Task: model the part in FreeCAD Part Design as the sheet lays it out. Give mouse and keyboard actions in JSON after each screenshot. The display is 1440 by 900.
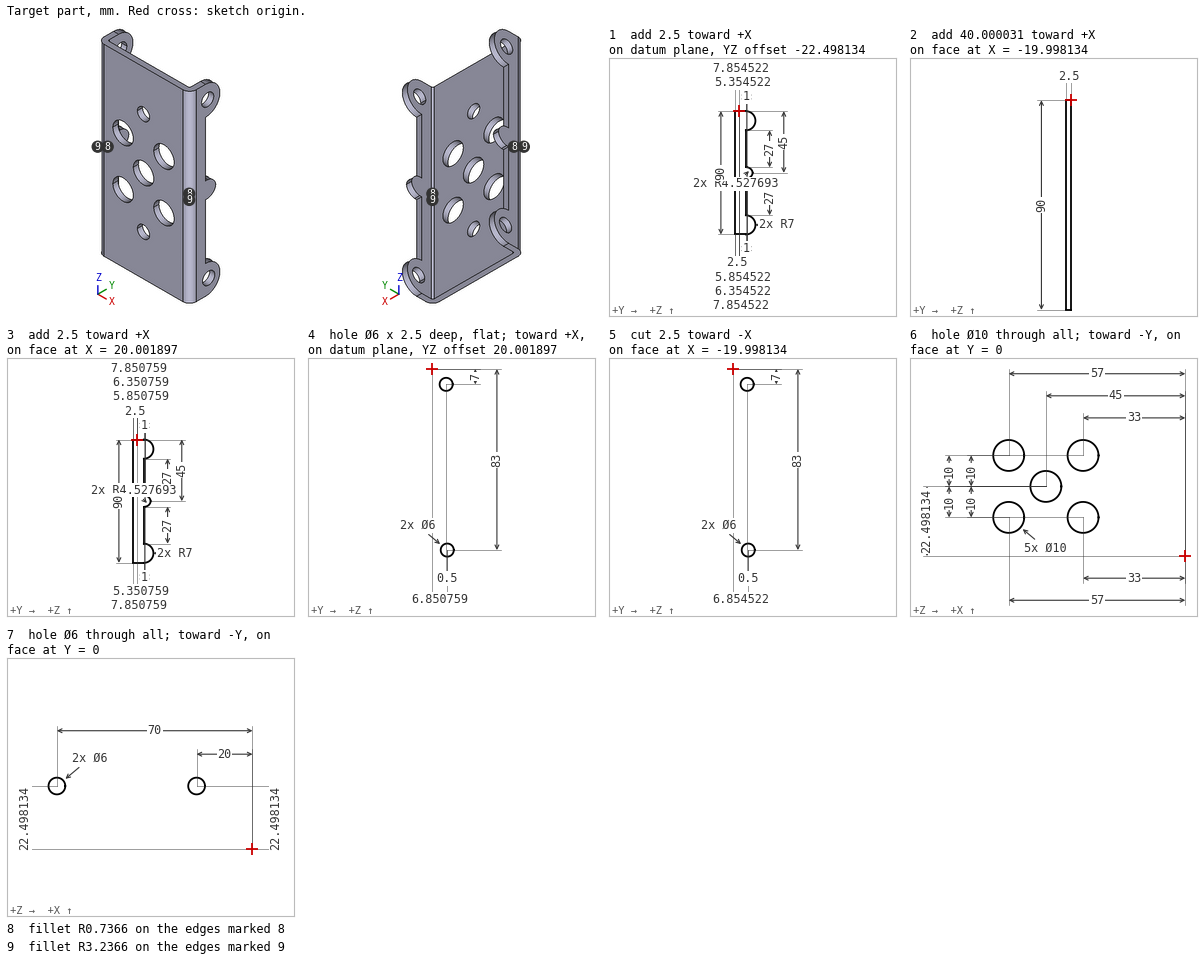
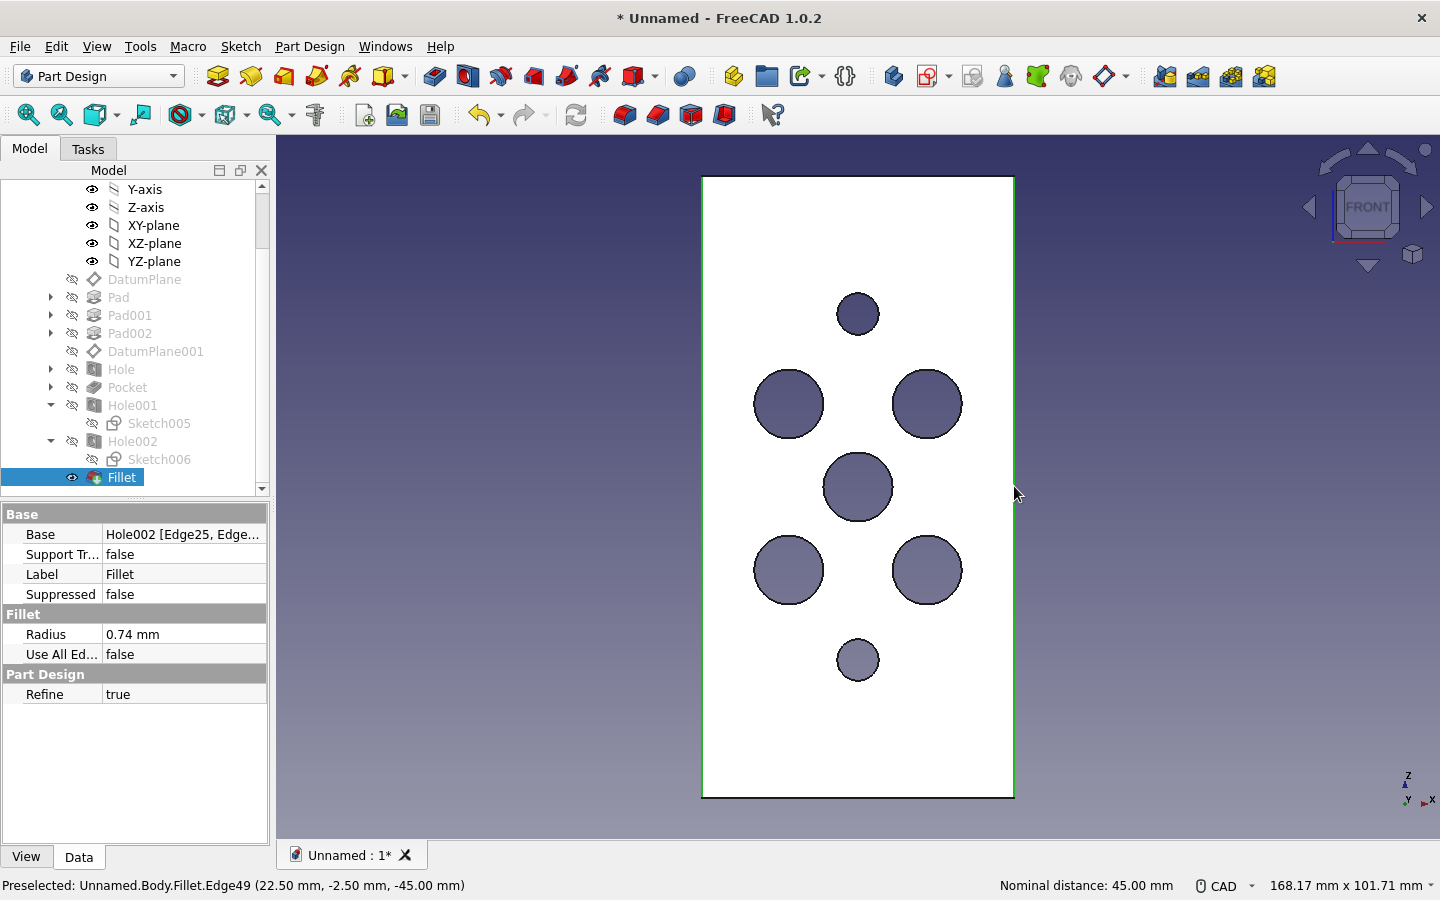
{"action": "left_click", "coordinate": [625, 116]}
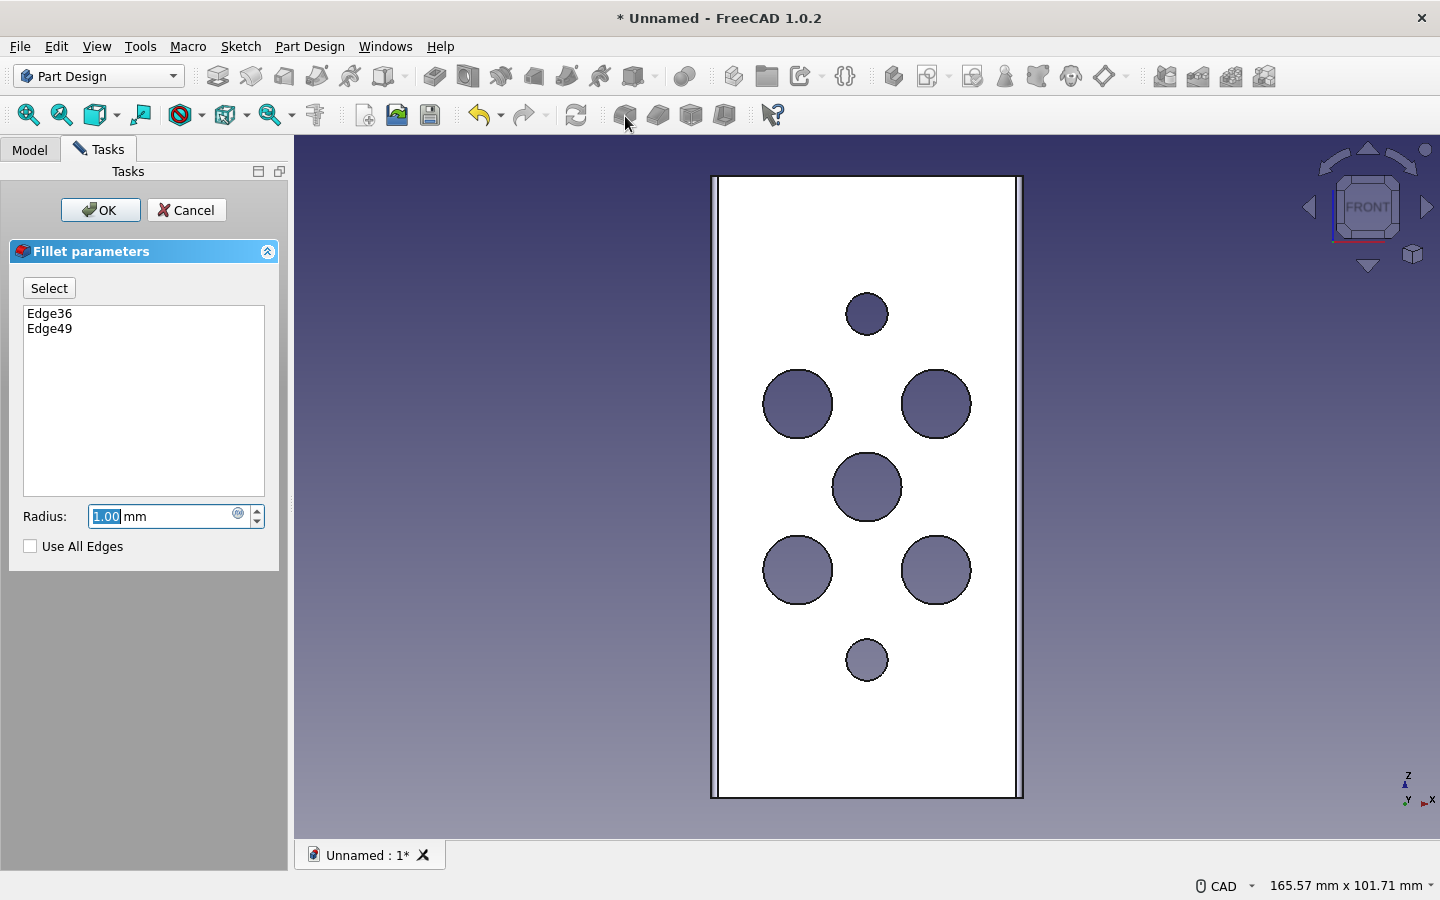
{"action": "type", "text": "3.2366"}
{"action": "key", "text": "Tab"}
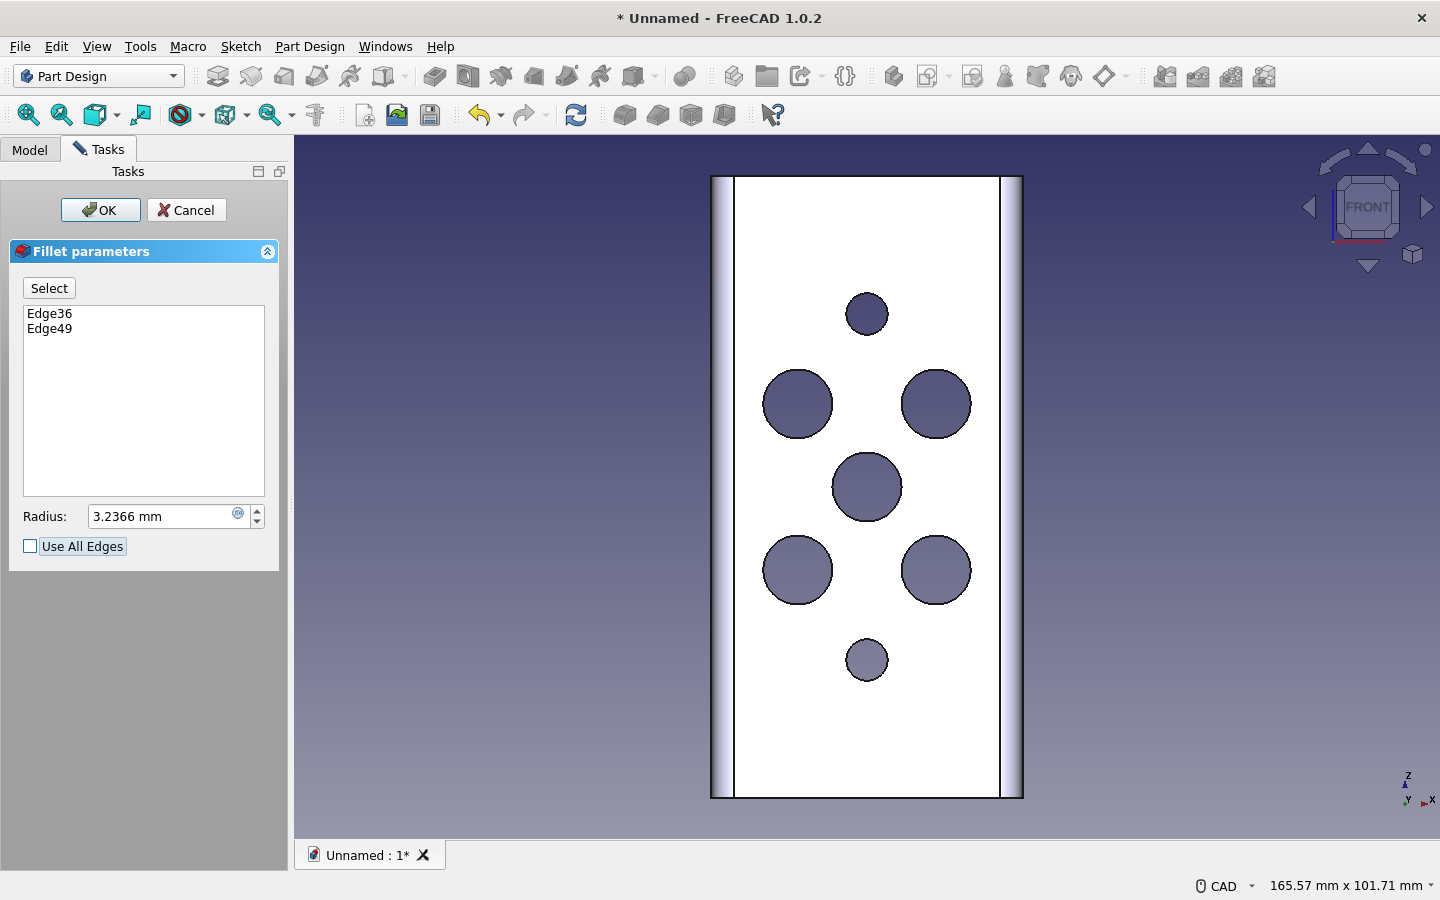
{"action": "left_click", "coordinate": [101, 210]}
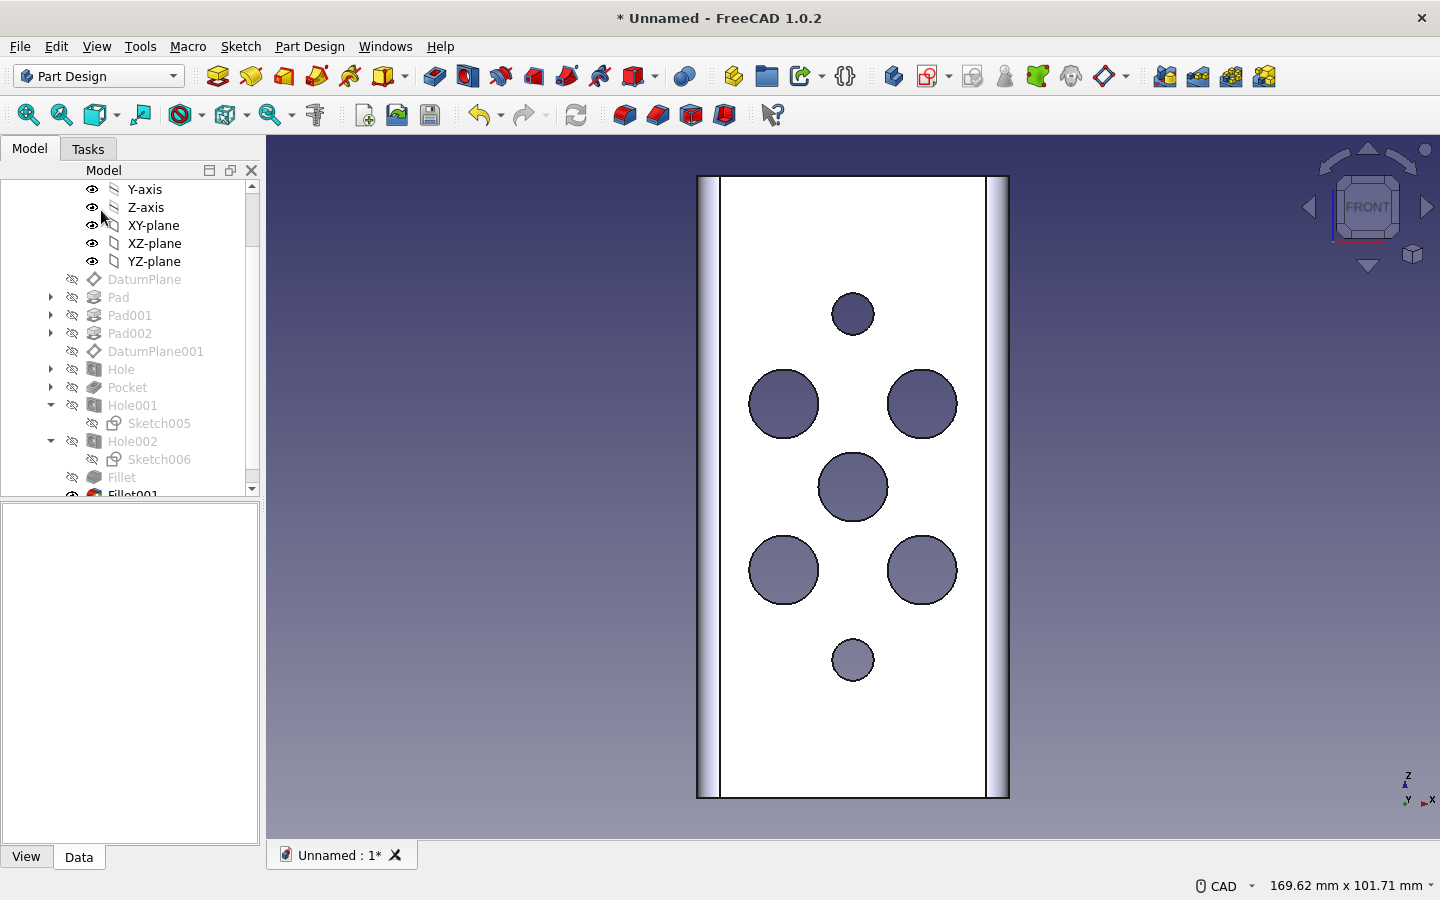
{"action": "key", "text": "0"}